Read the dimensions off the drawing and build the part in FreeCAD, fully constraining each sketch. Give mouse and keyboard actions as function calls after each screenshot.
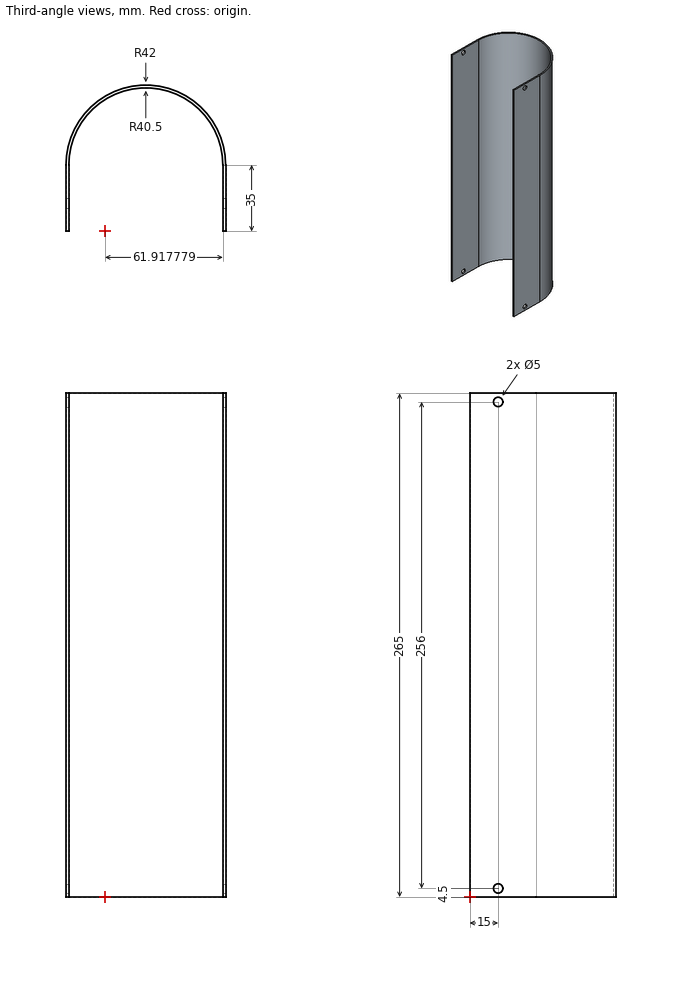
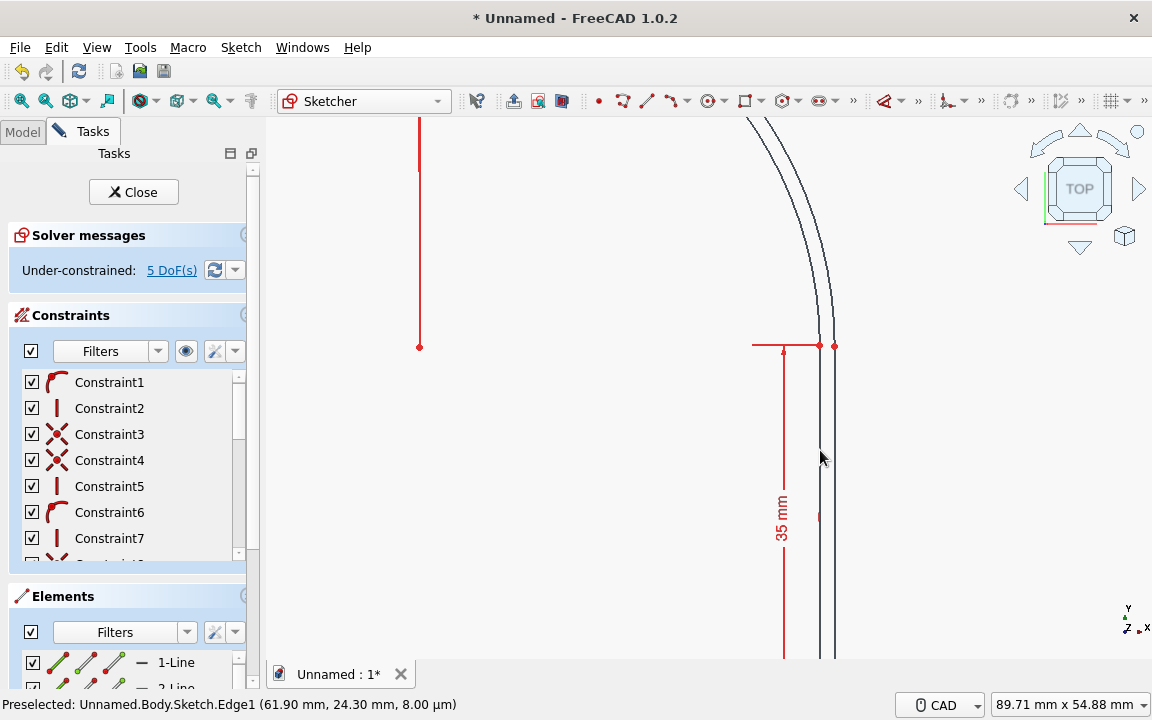
click(835, 588)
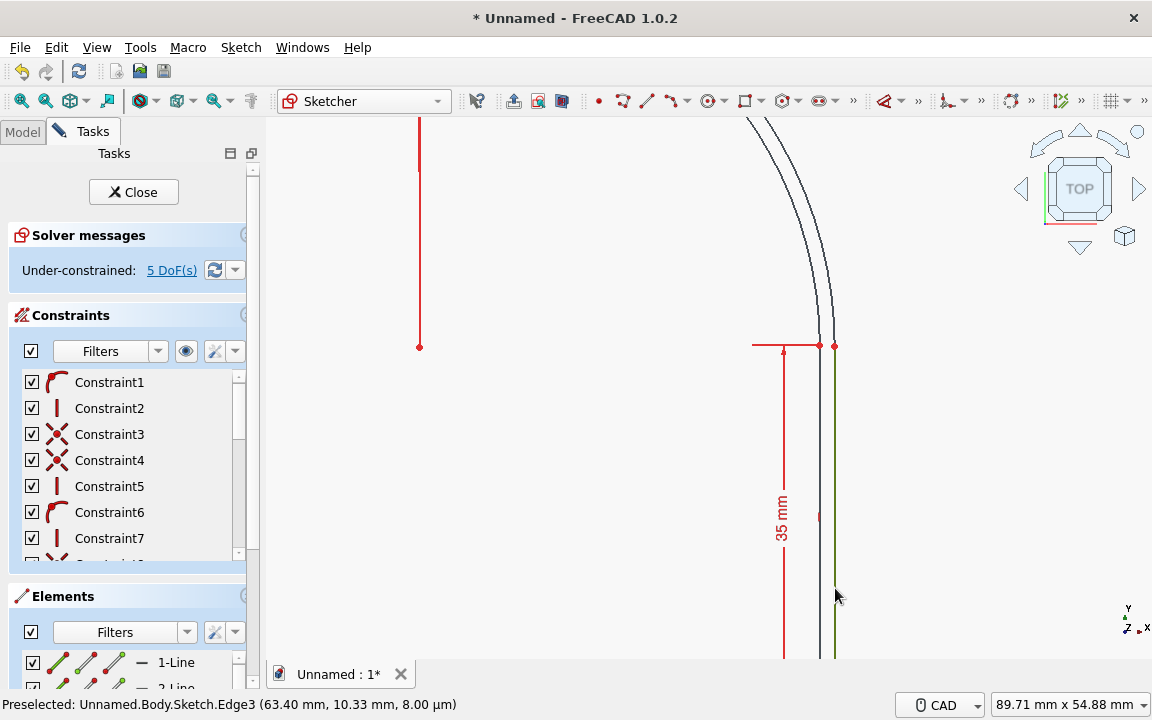
key(i)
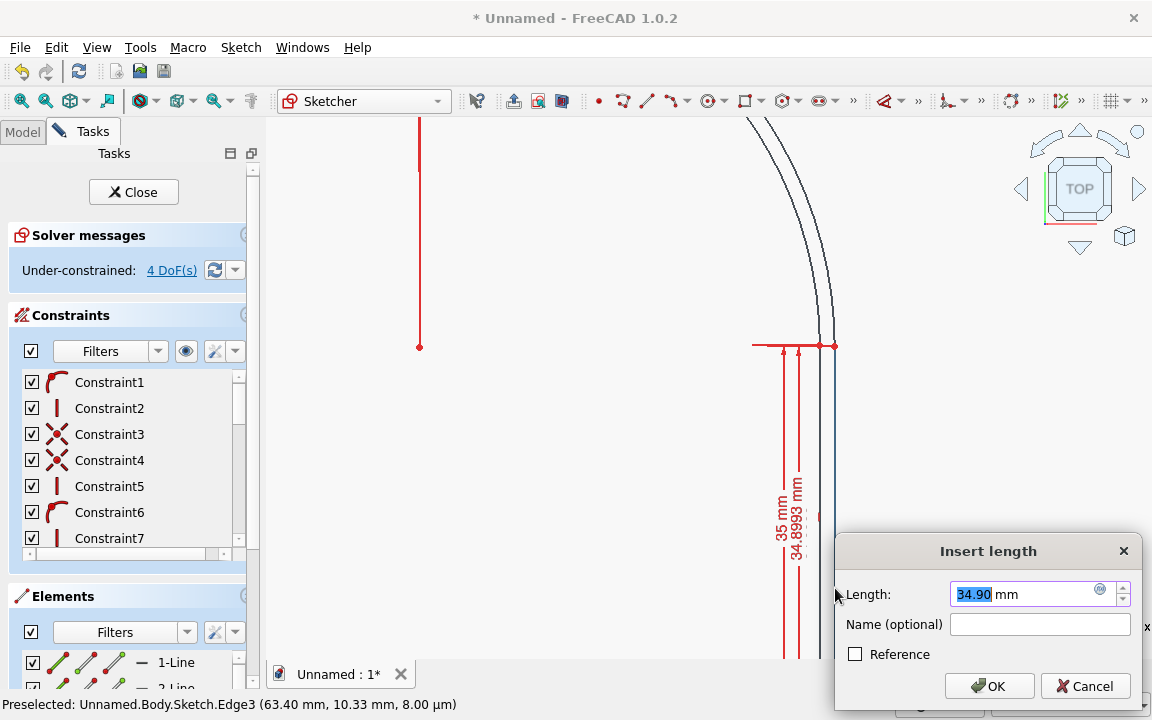
text(35)
key(Return)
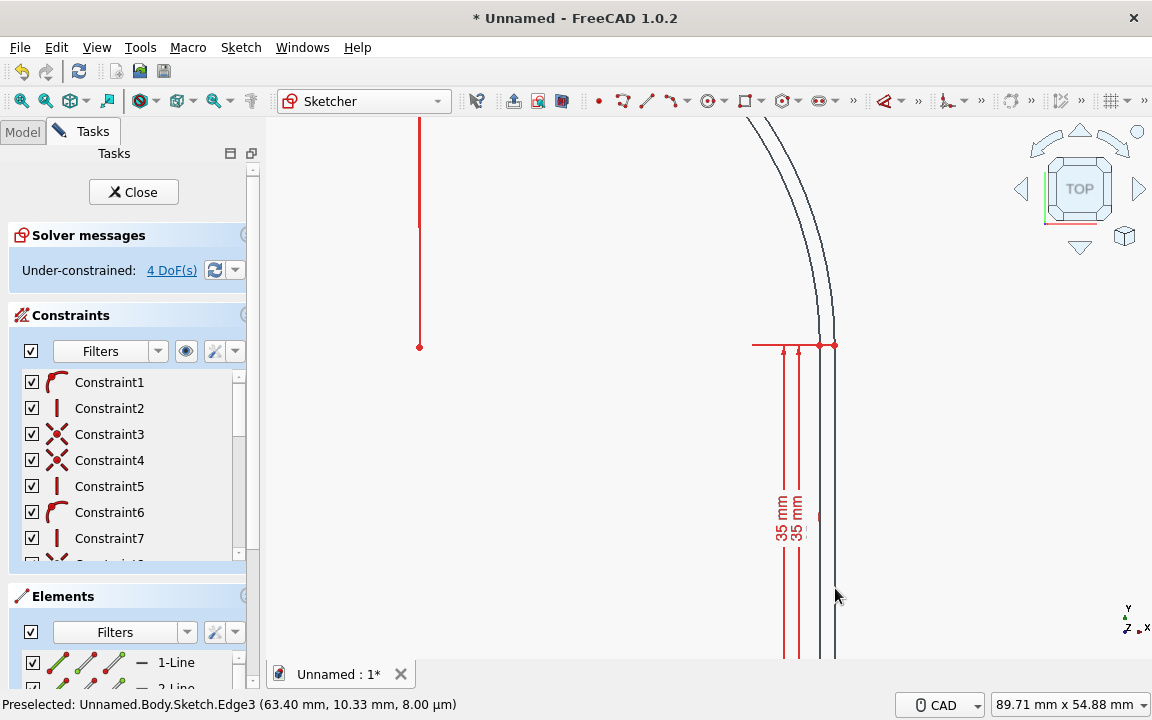
scroll(820, 451, down, 4)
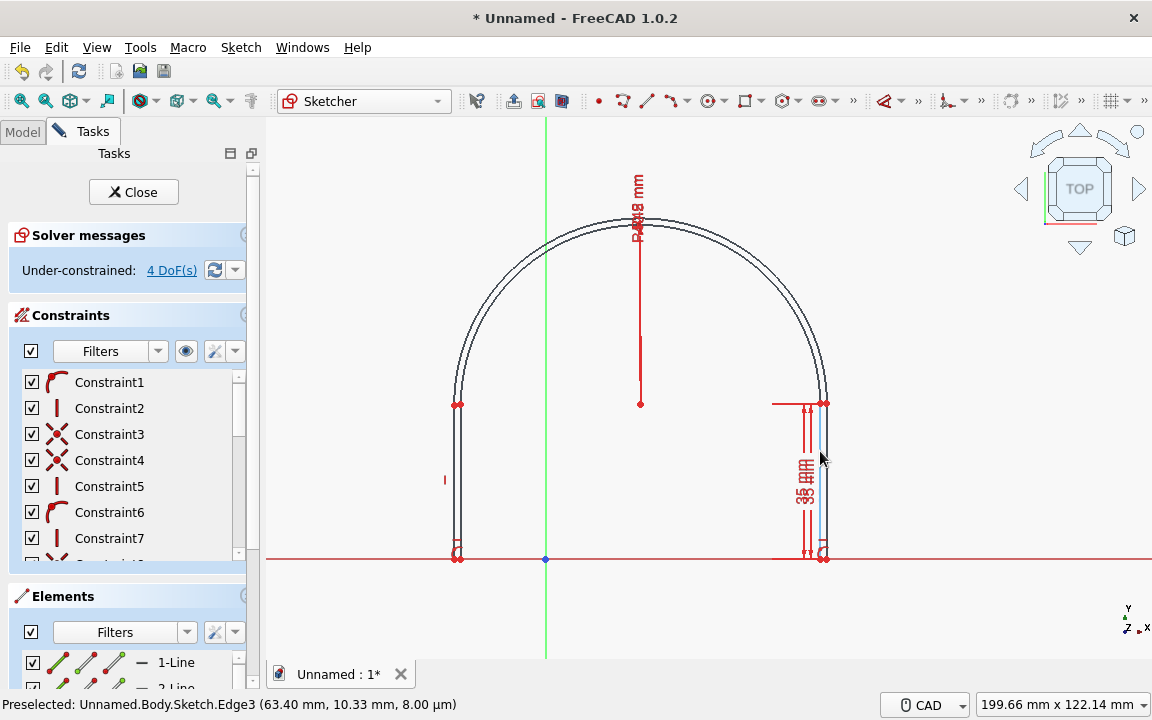
scroll(454, 451, up, 4)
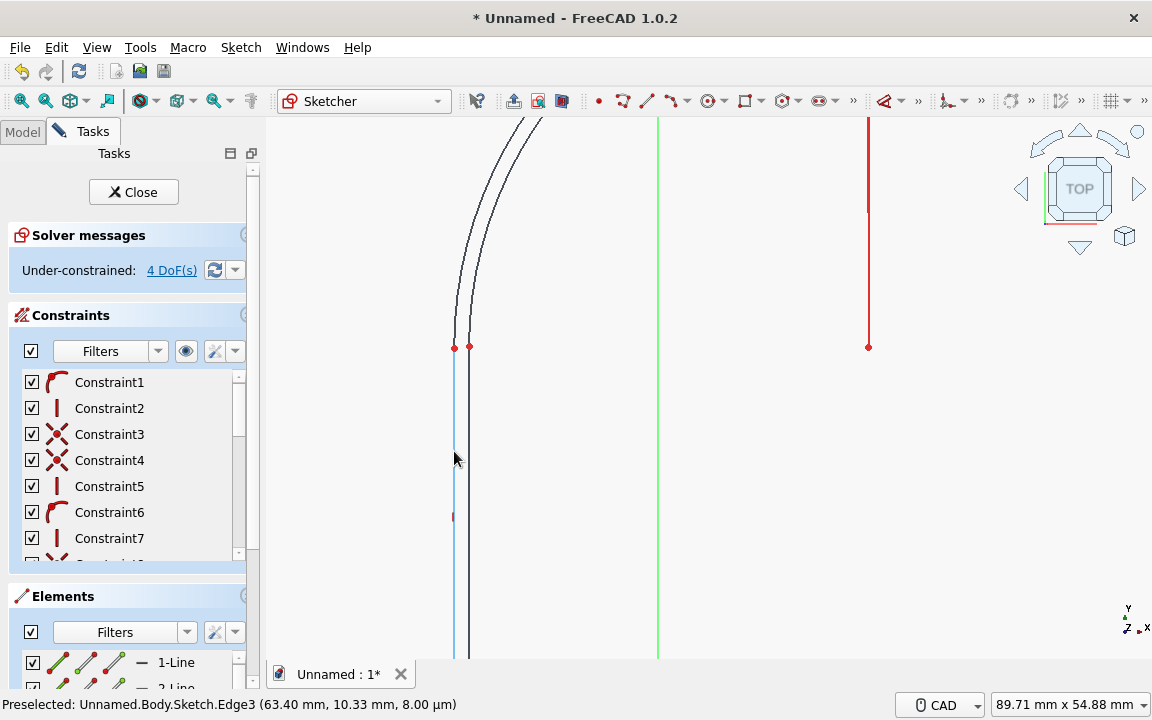
click(454, 451)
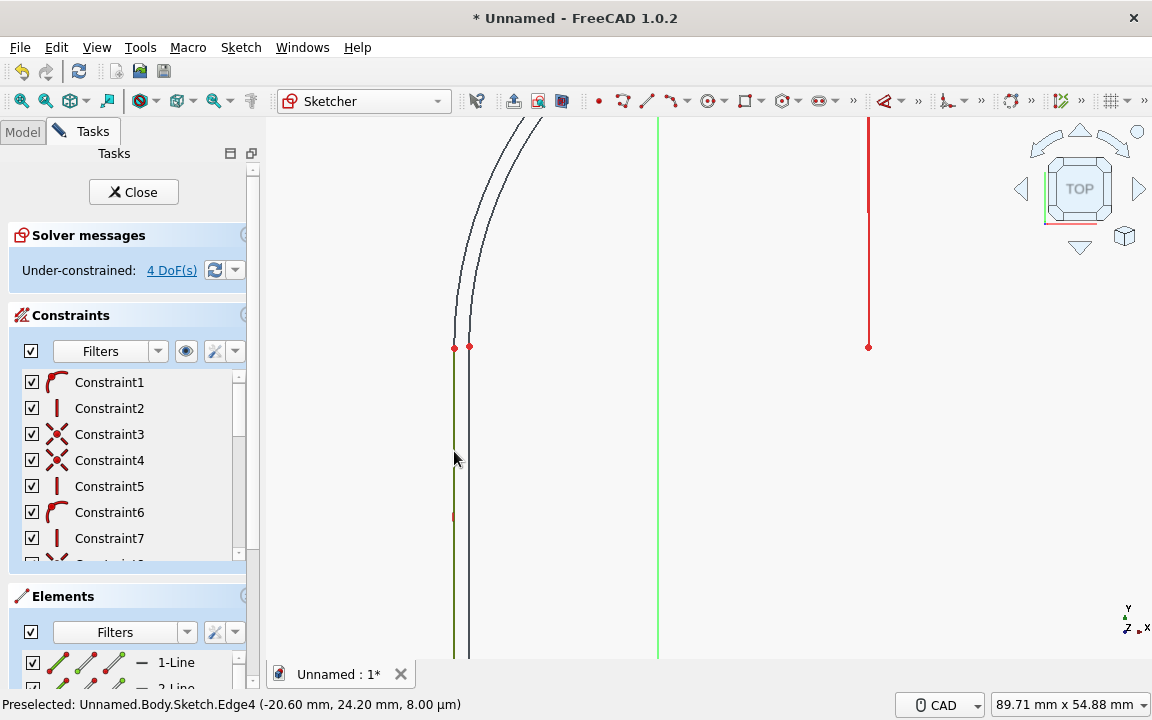
key(i)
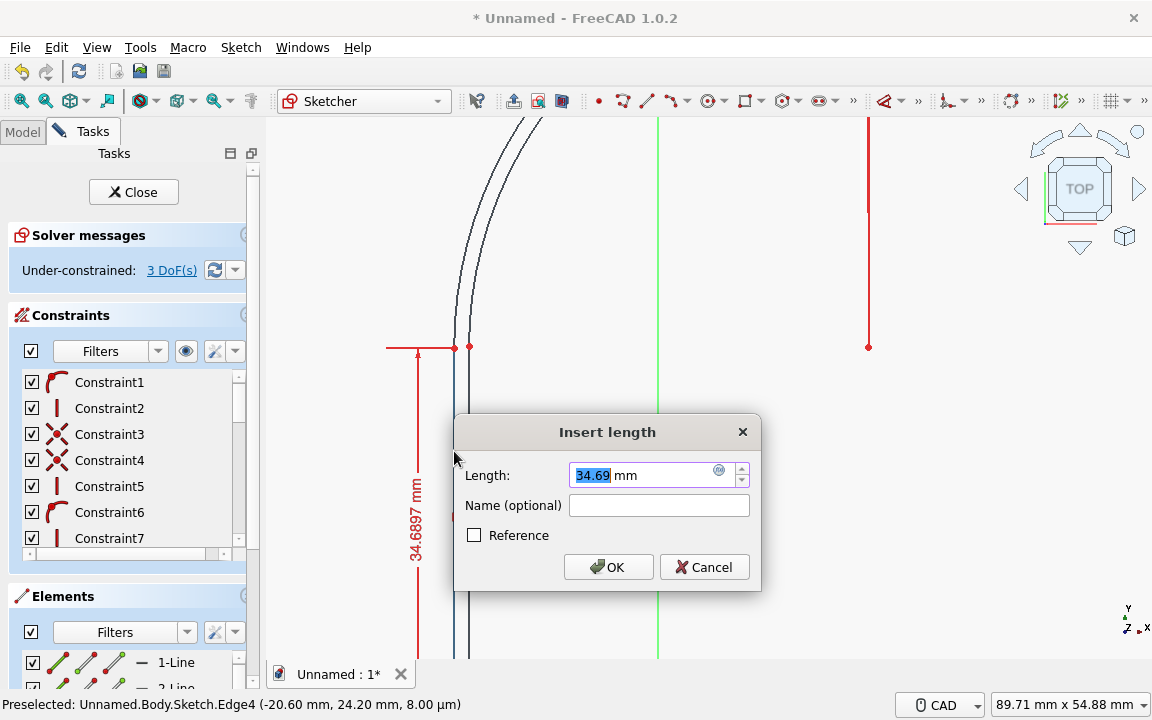
text(35)
key(Return)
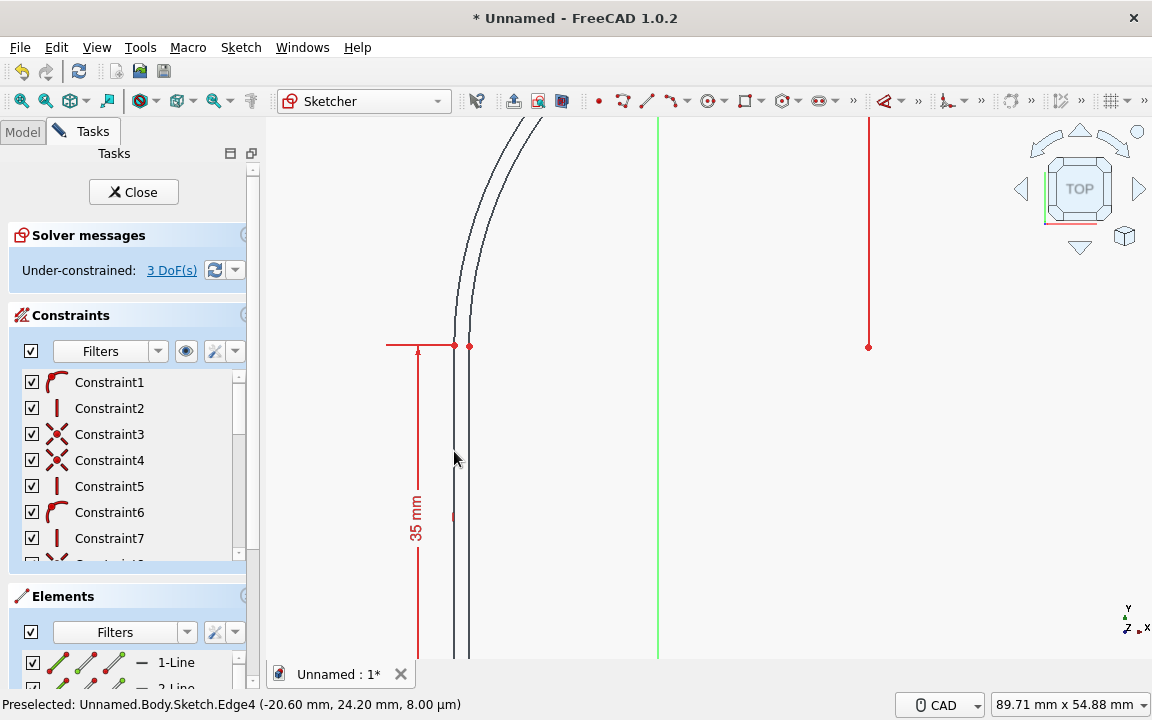
click(469, 588)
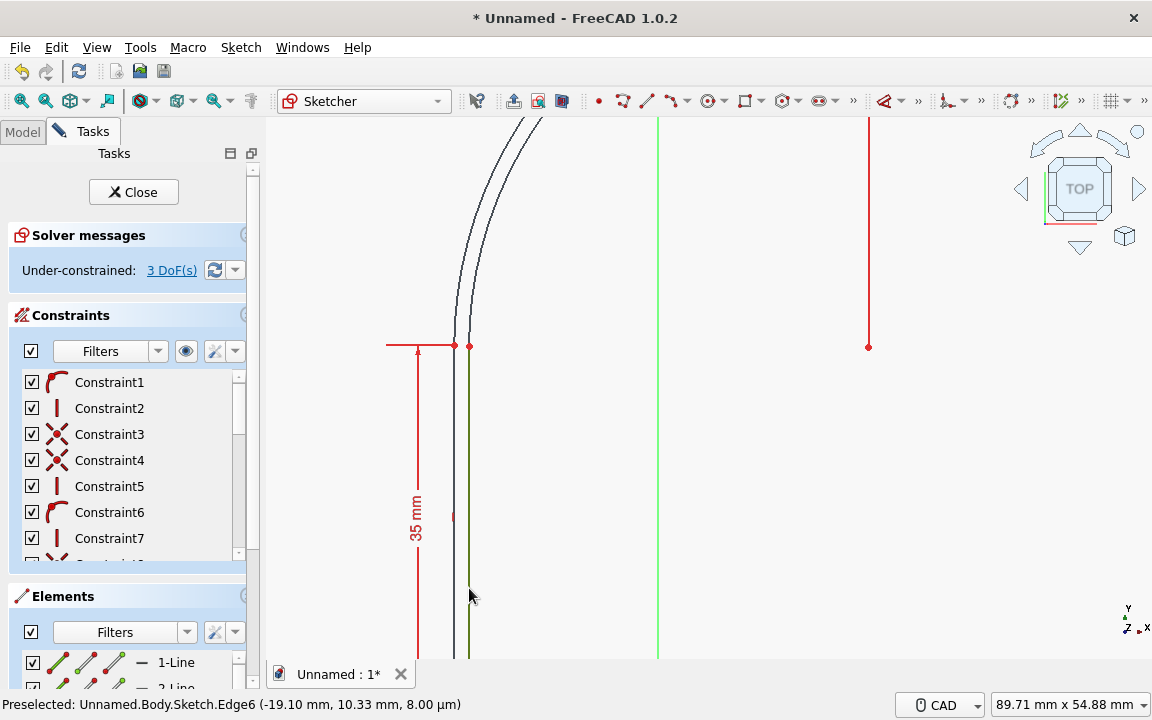
click(904, 102)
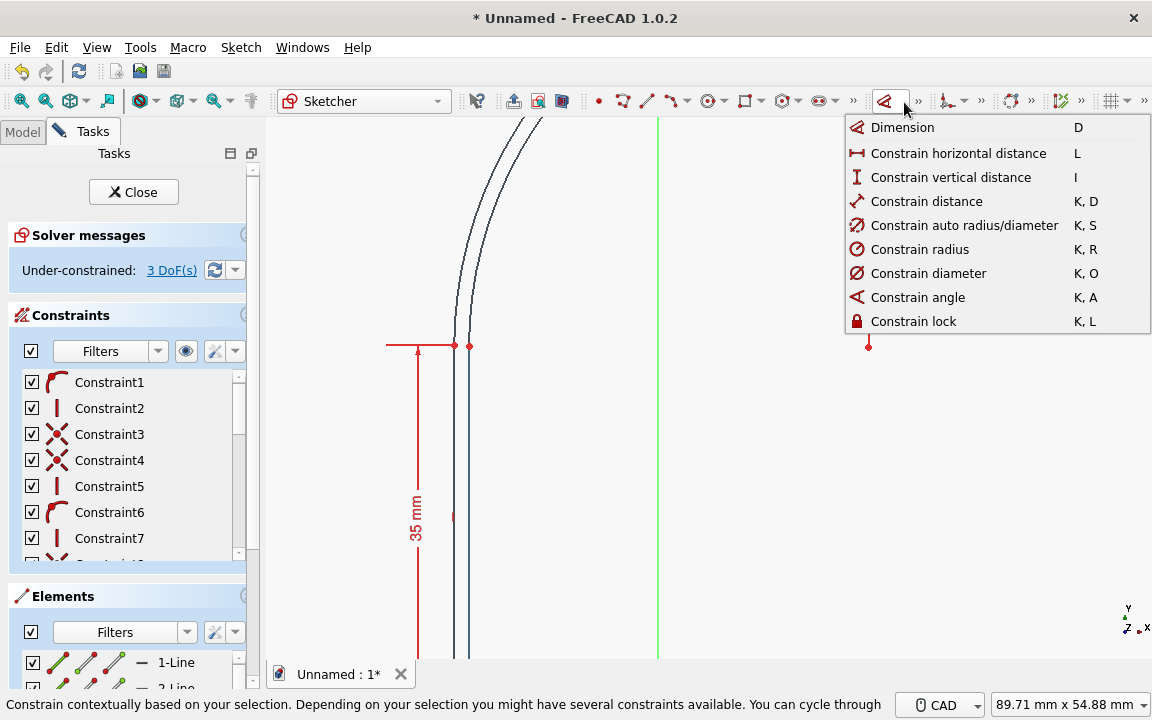
click(998, 177)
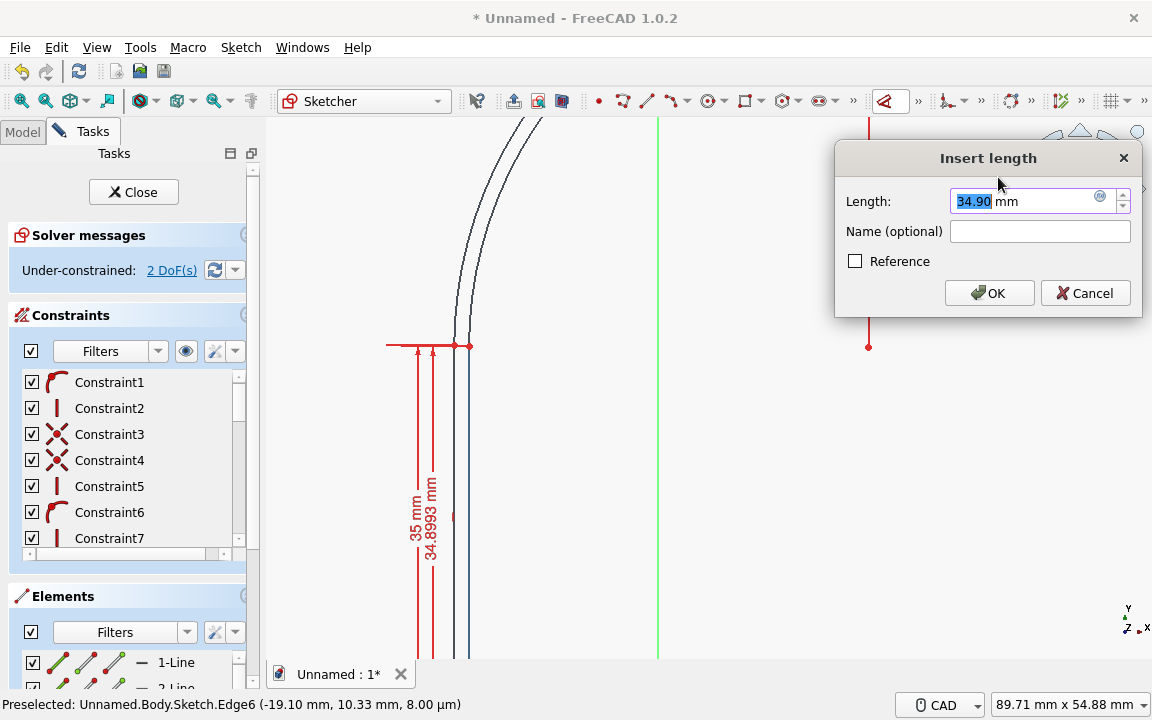
text(35)
key(Return)